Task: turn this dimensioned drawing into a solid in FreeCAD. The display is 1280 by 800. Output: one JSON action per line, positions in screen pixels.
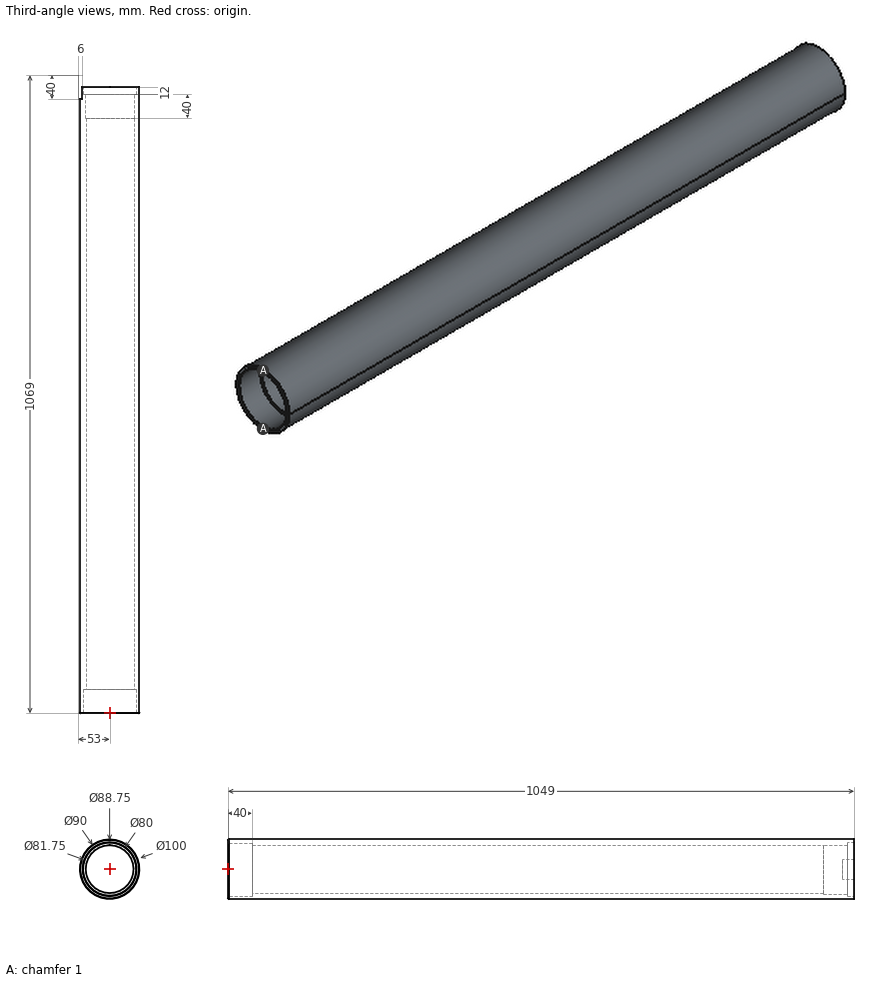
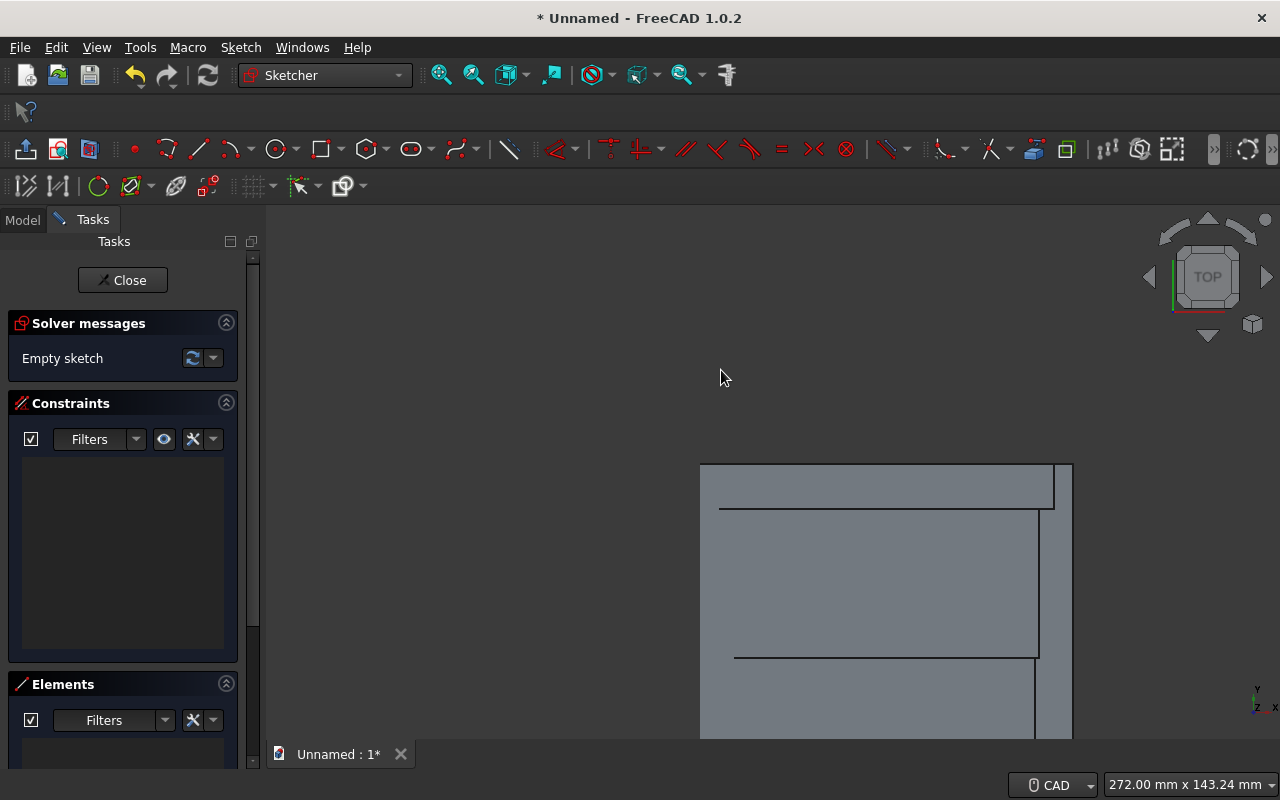
{"action": "scroll", "coordinate": [696, 457], "scroll_direction": "up", "scroll_amount": 4}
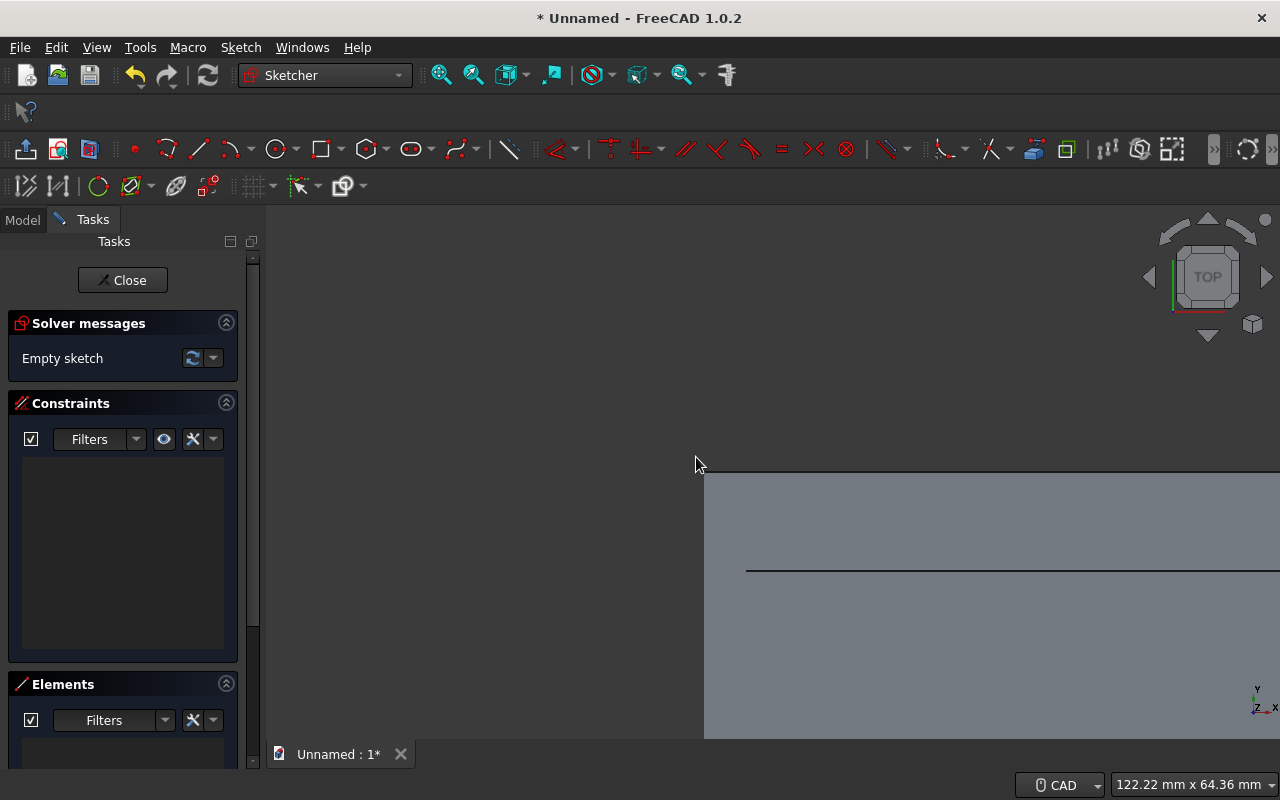
{"action": "left_click", "coordinate": [322, 150]}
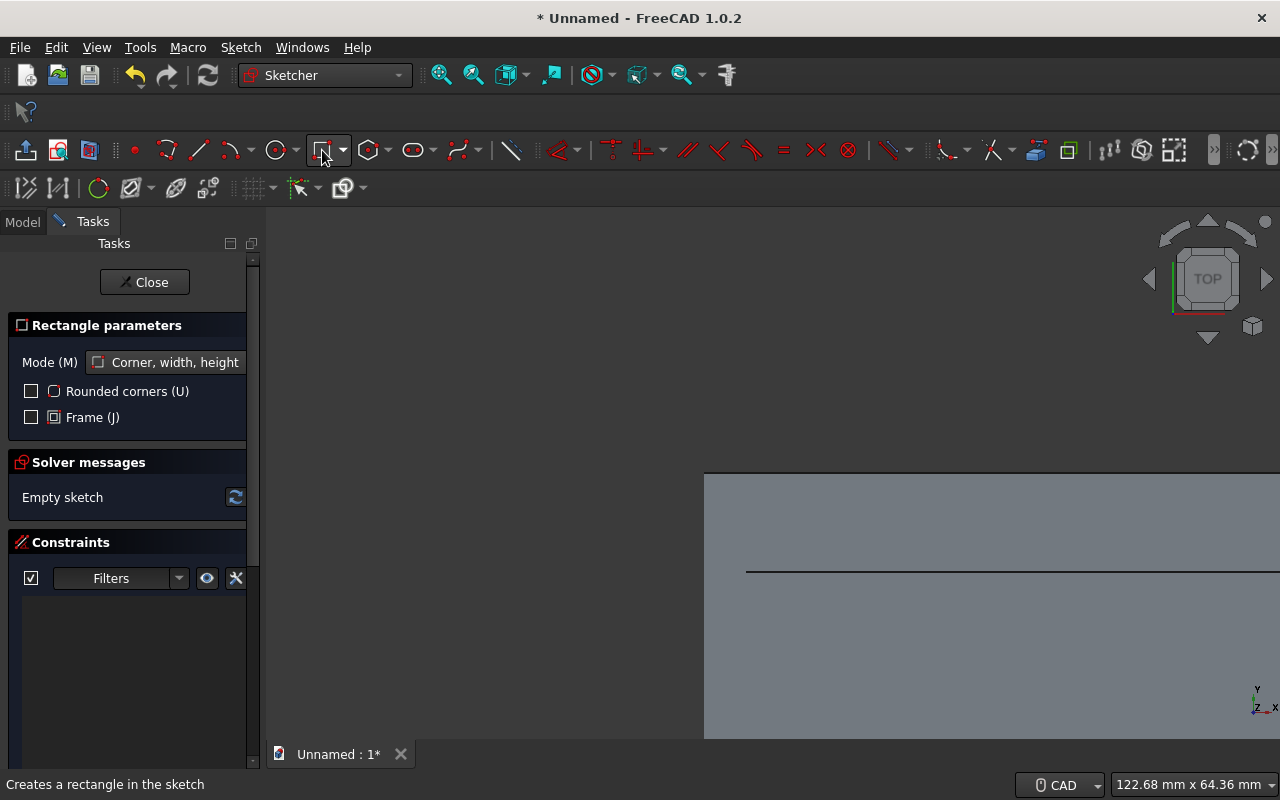
{"action": "left_click", "coordinate": [680, 307]}
{"action": "mouse_move", "coordinate": [729, 638]}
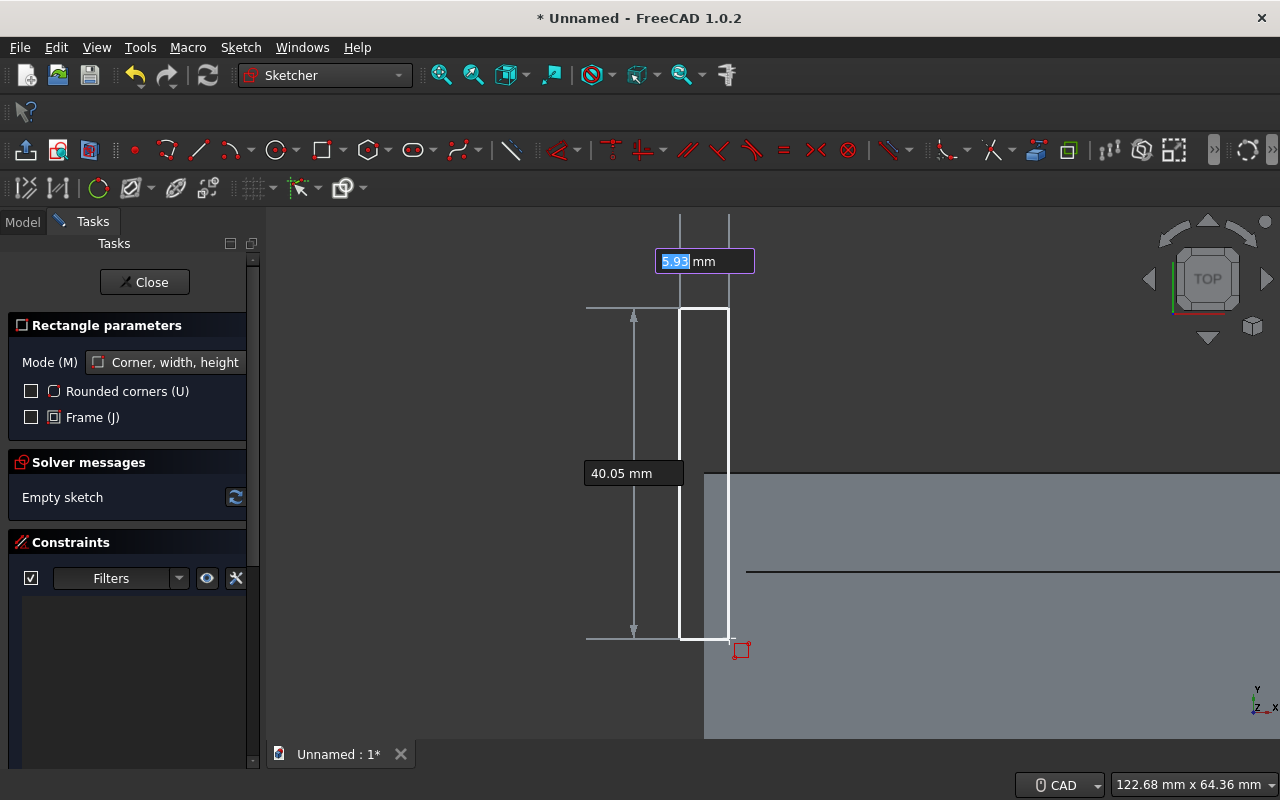
{"action": "type", "text": "6"}
{"action": "key", "text": "Tab"}
{"action": "type", "text": "40"}
{"action": "key", "text": "Return"}
{"action": "key", "text": "Escape"}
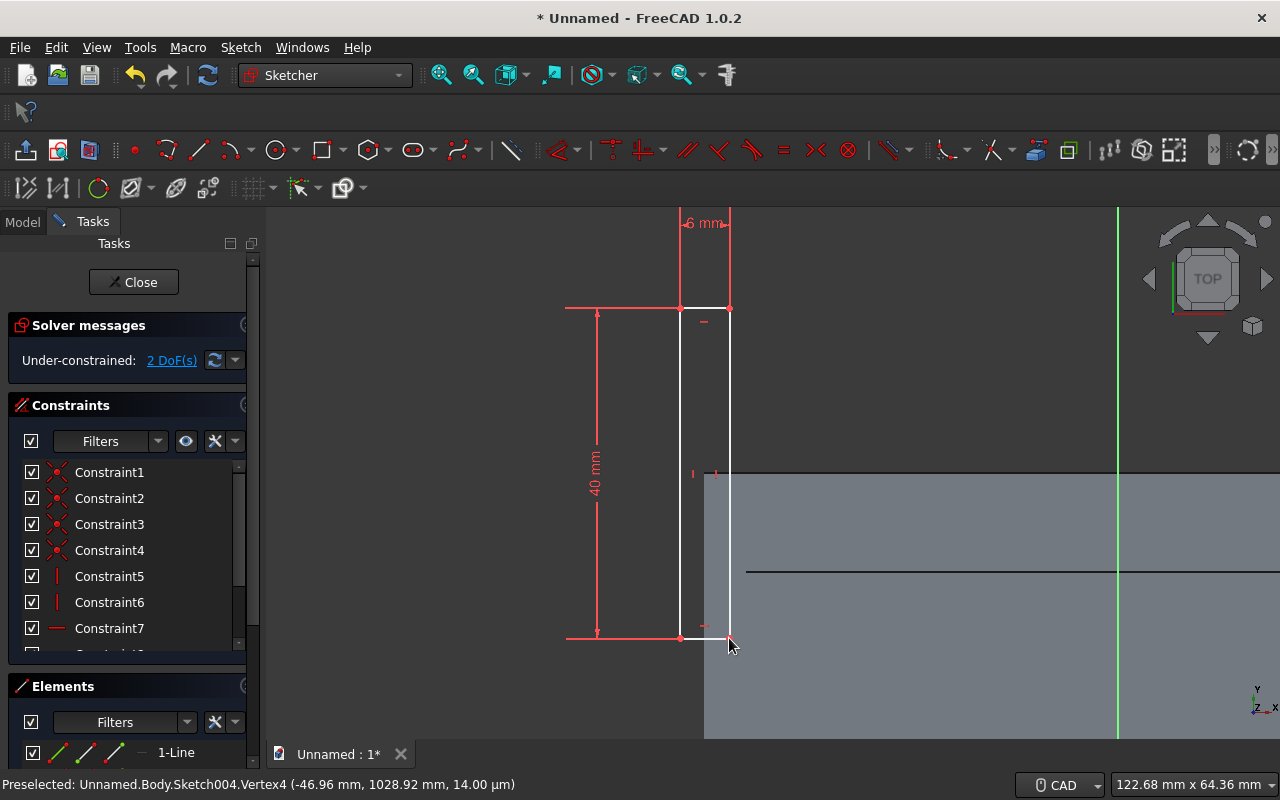
{"action": "left_click", "coordinate": [558, 150]}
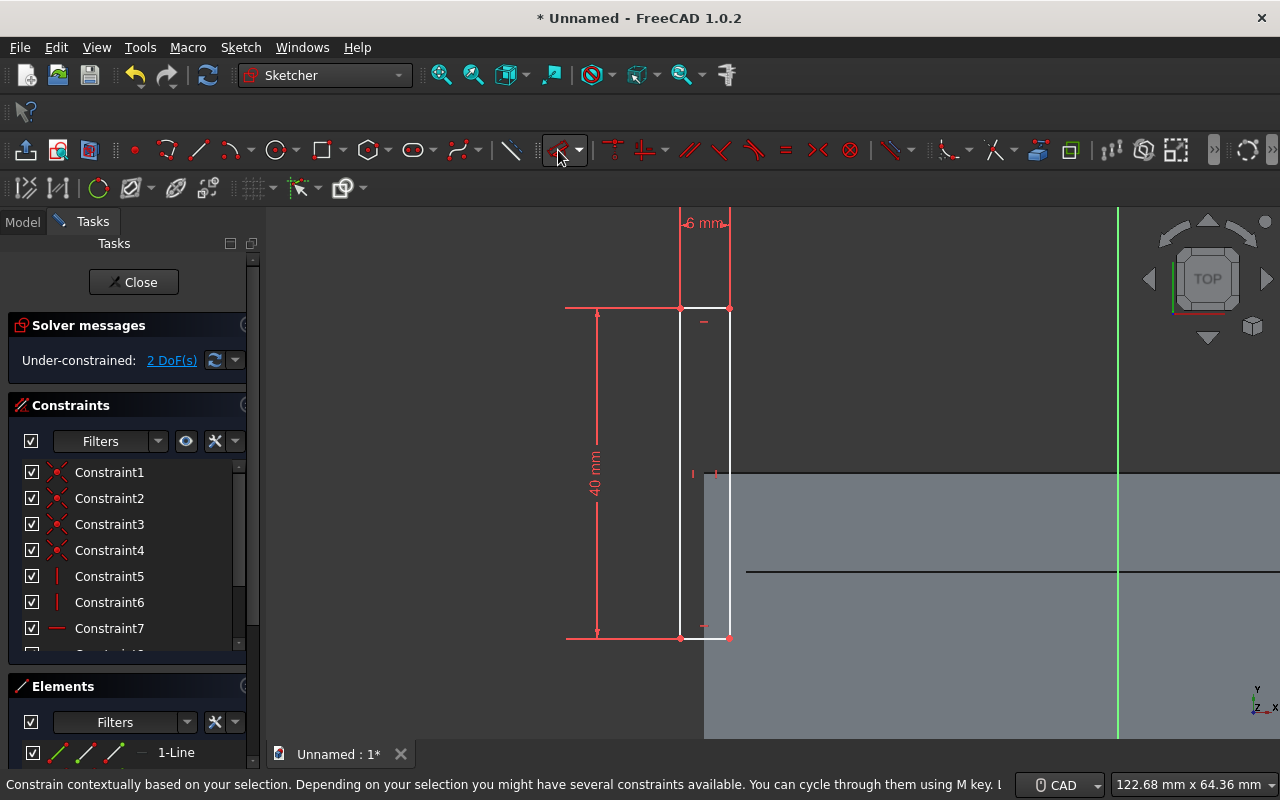
{"action": "left_click", "coordinate": [680, 308]}
{"action": "left_click", "coordinate": [898, 274]}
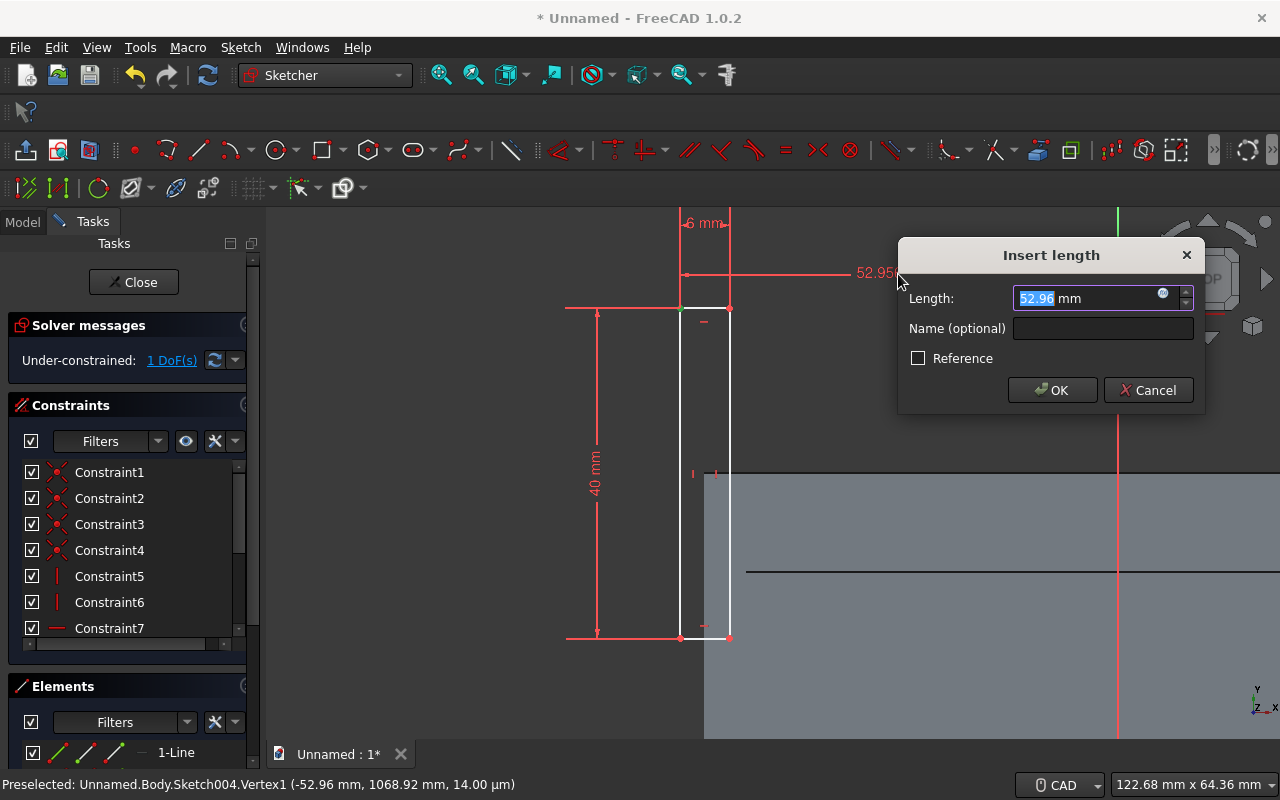
{"action": "type", "text": "53"}
{"action": "key", "text": "Return"}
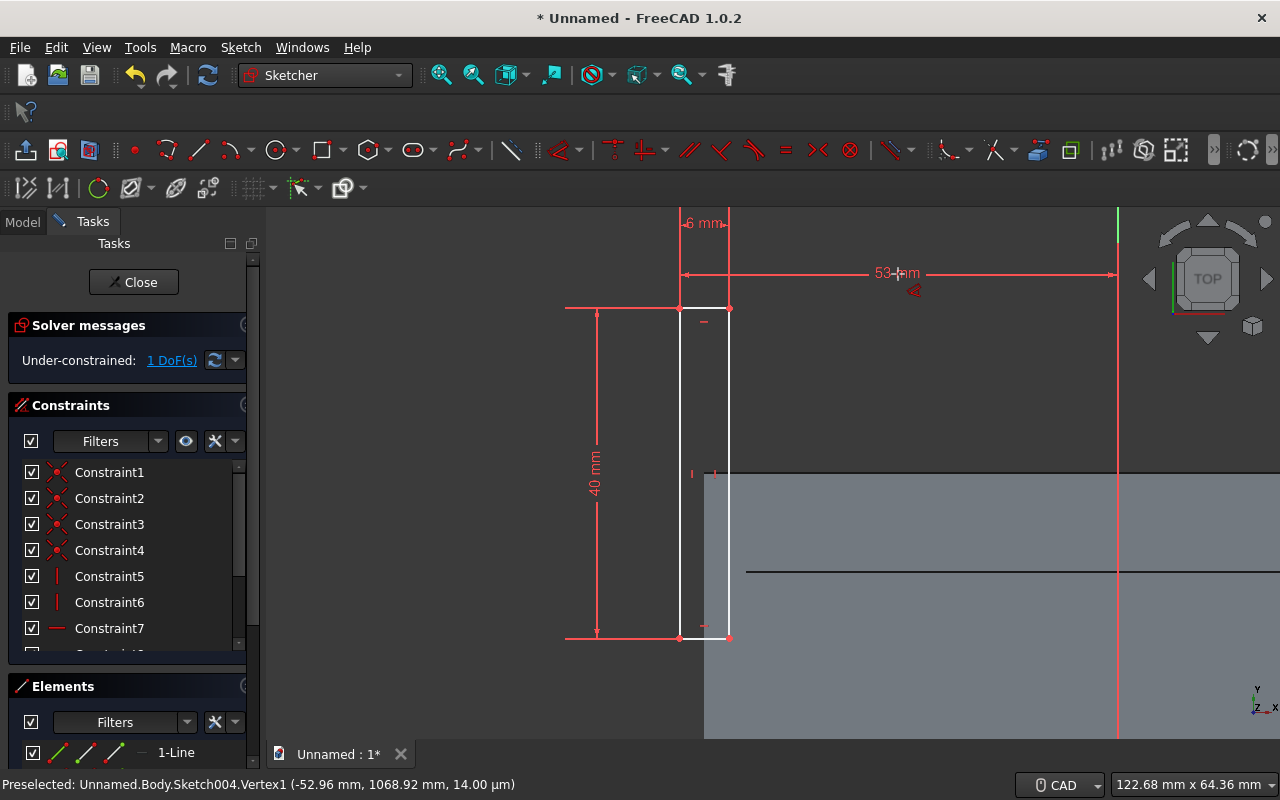
{"action": "left_click", "coordinate": [680, 308]}
{"action": "left_click", "coordinate": [646, 509]}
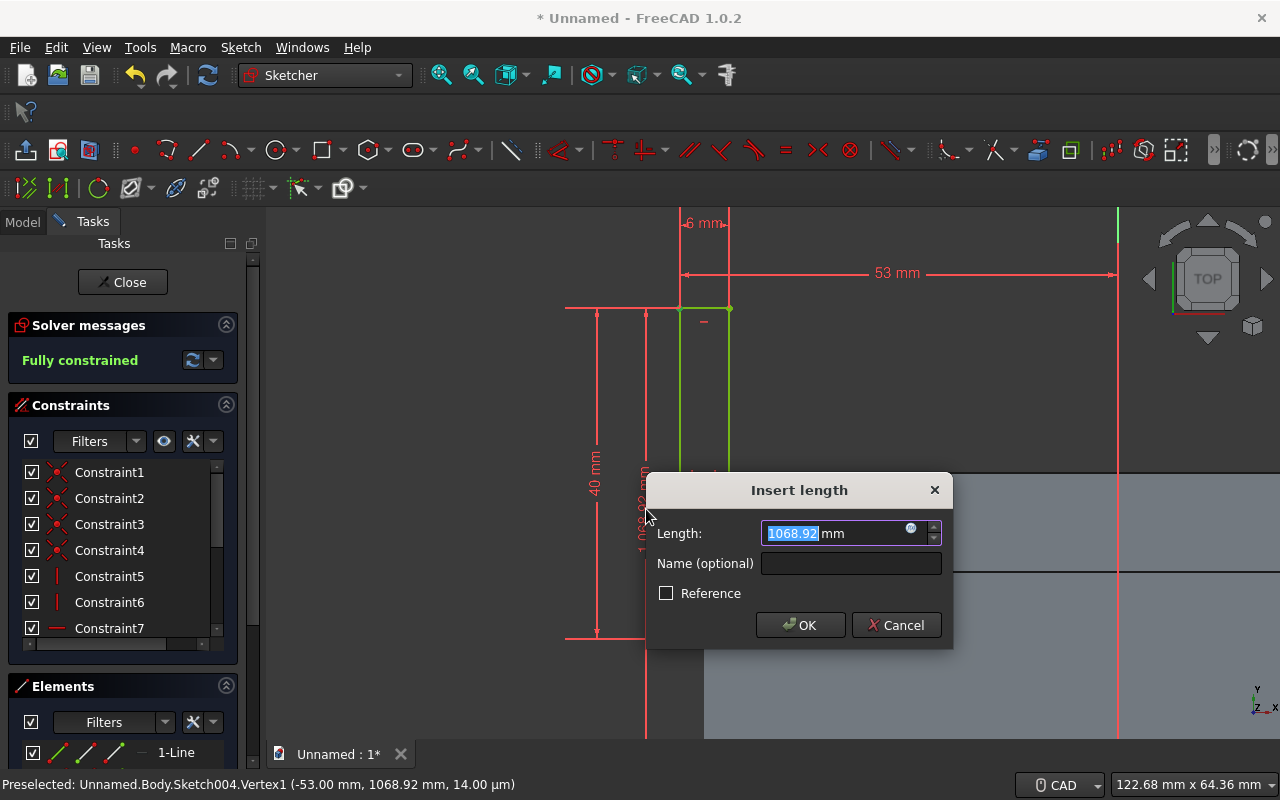
{"action": "type", "text": "1069"}
{"action": "key", "text": "Return"}
{"action": "key", "text": "Escape"}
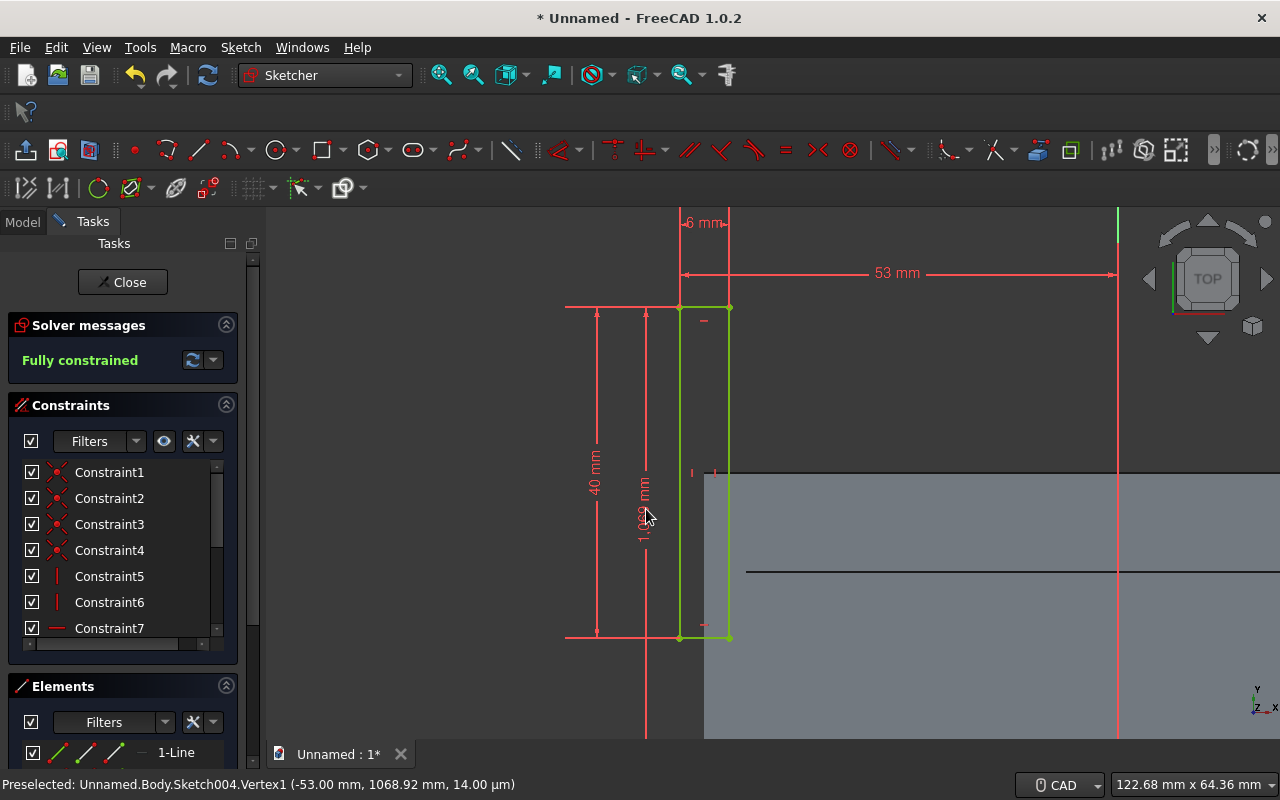
{"action": "left_click", "coordinate": [123, 282]}